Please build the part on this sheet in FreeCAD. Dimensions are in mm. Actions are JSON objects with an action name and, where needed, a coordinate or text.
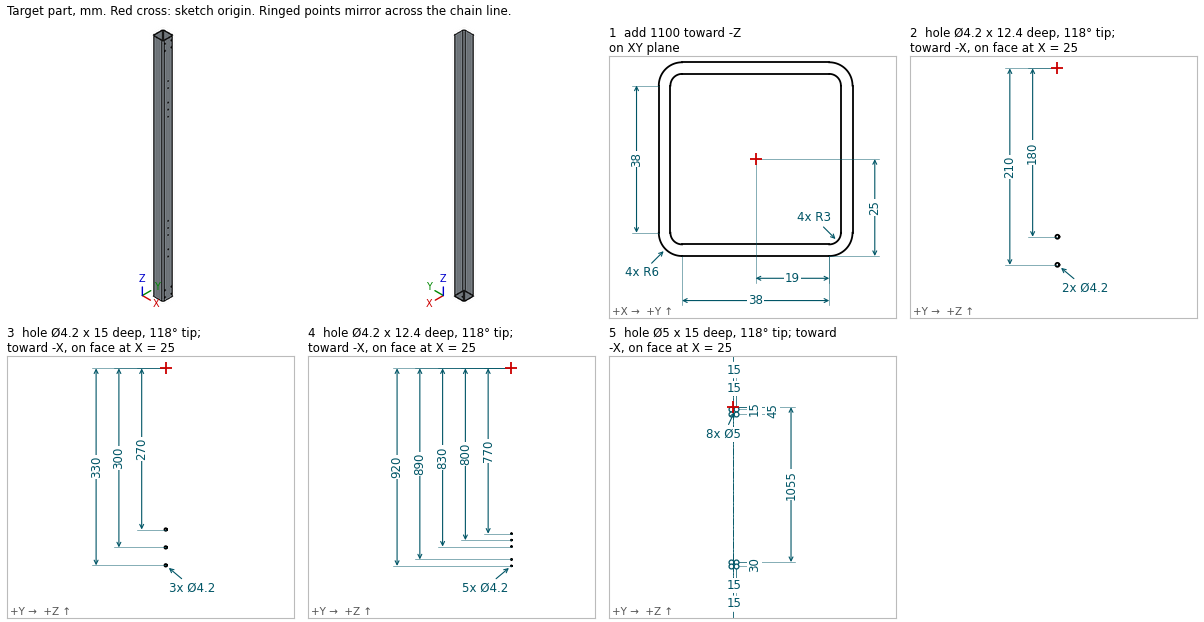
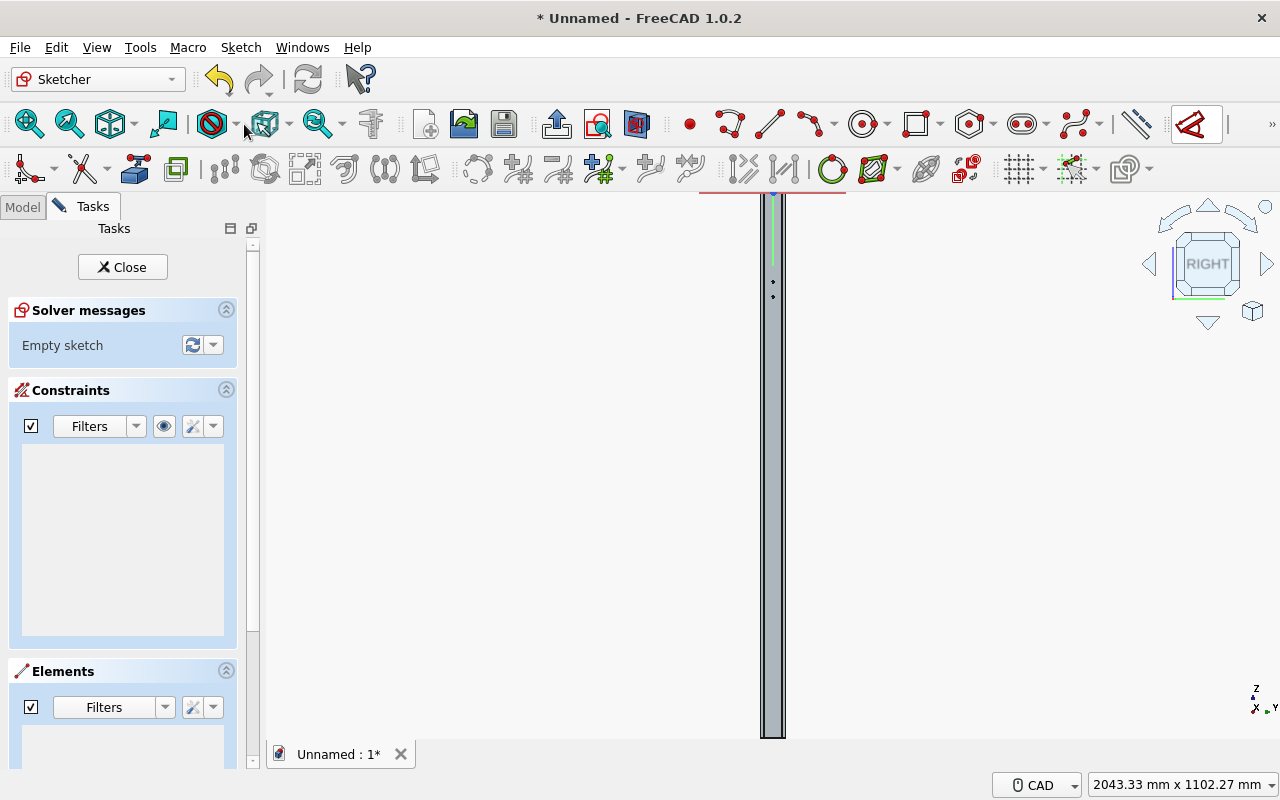
{"action": "scroll", "coordinate": [780, 329], "scroll_direction": "up", "scroll_amount": 12}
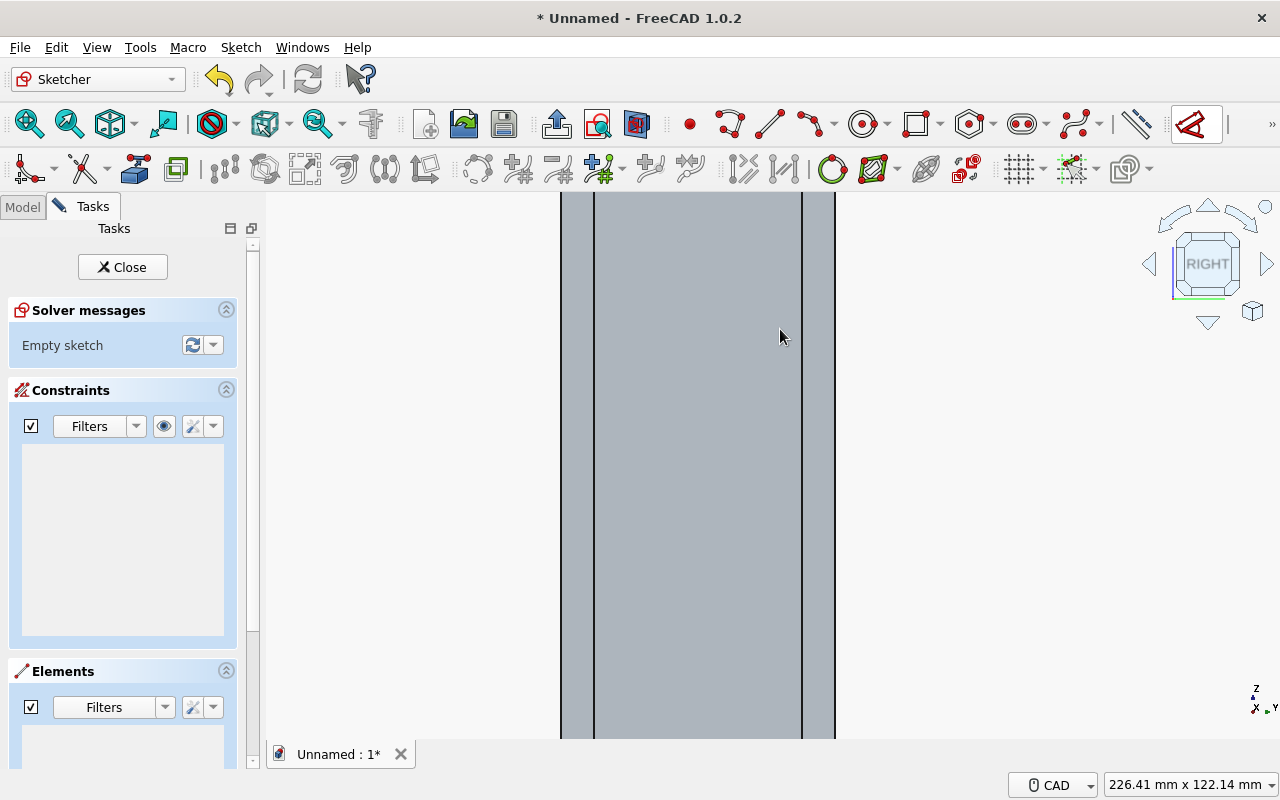
{"action": "left_click", "coordinate": [864, 124]}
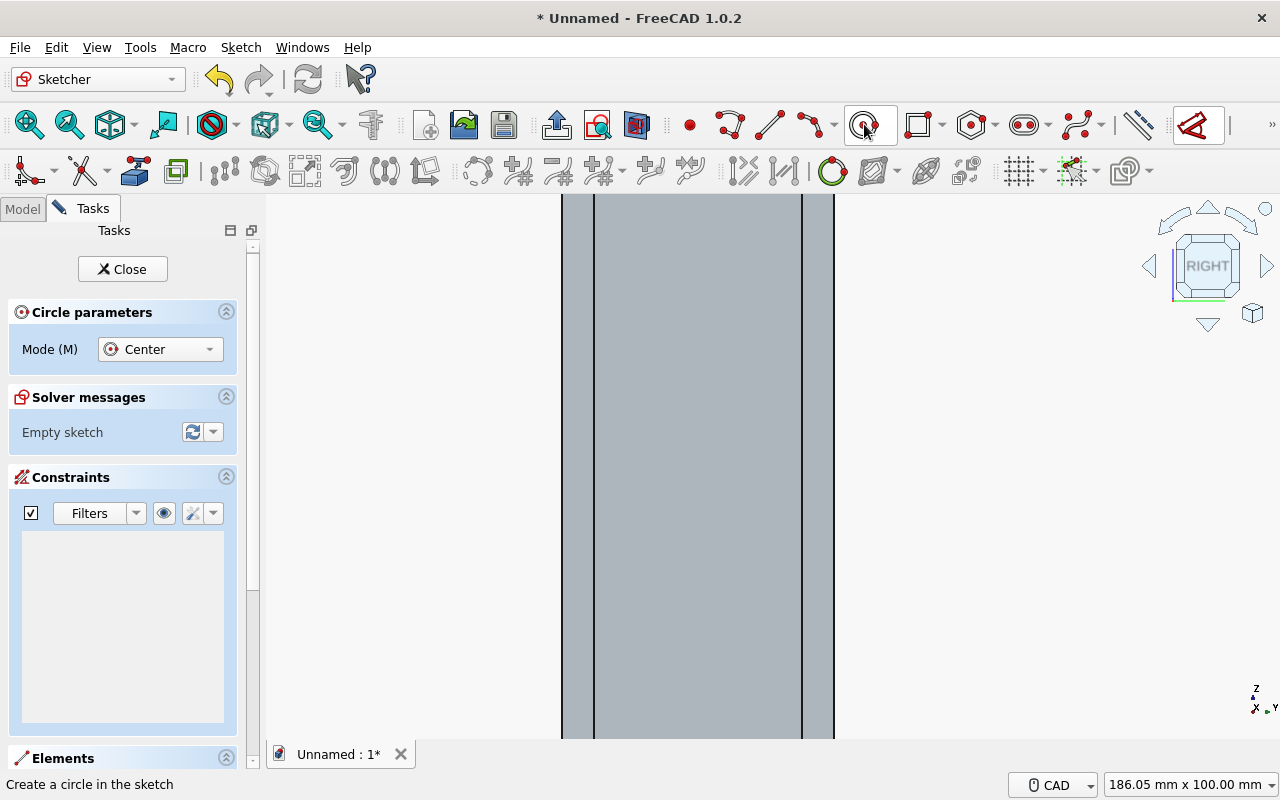
{"action": "scroll", "coordinate": [698, 301], "scroll_direction": "up", "scroll_amount": 4}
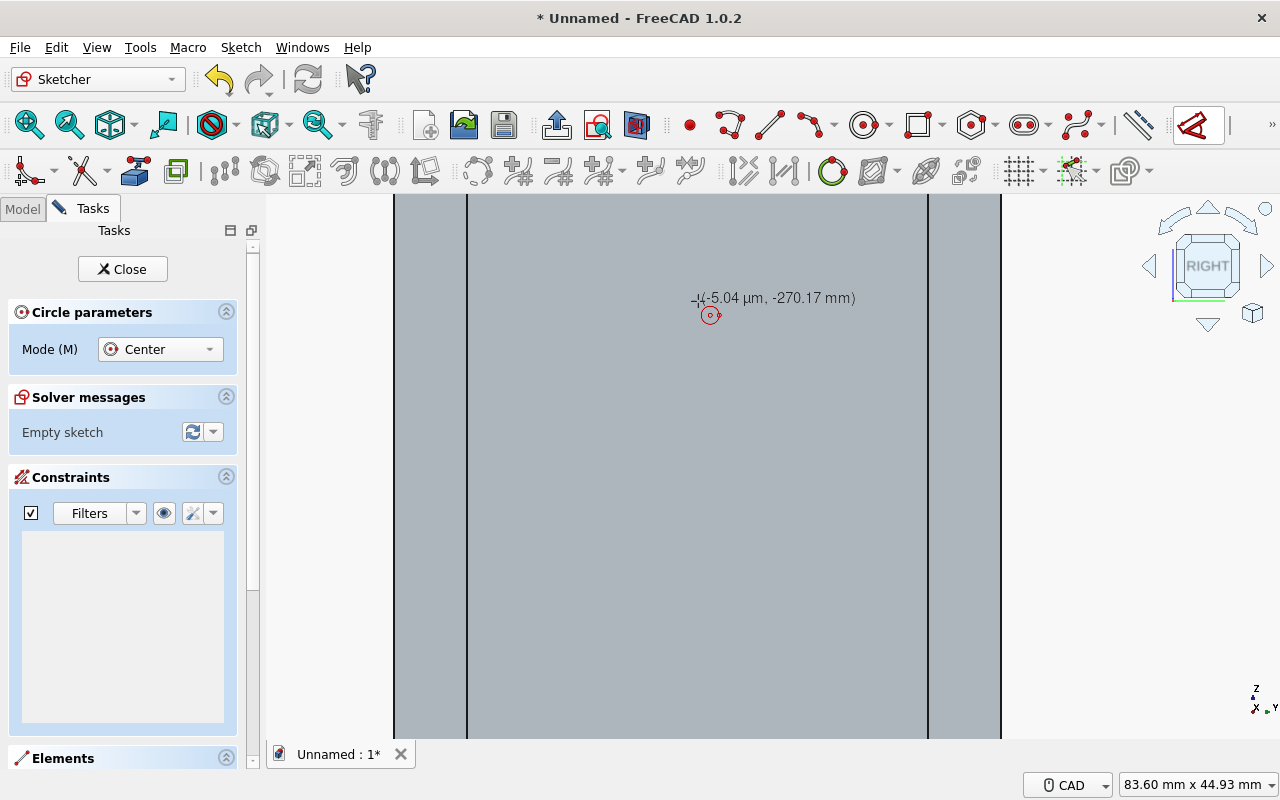
{"action": "left_click", "coordinate": [698, 301]}
{"action": "mouse_move", "coordinate": [716, 283]}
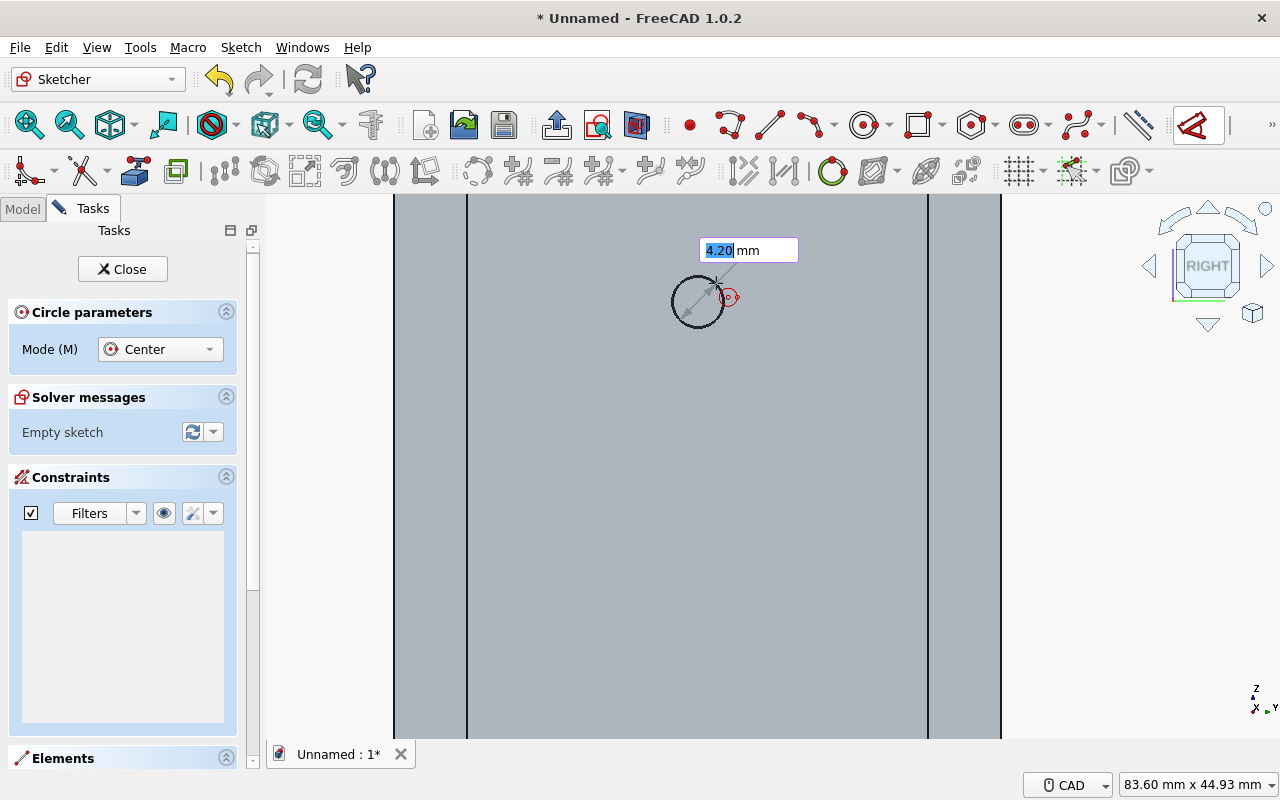
{"action": "type", "text": "4.2"}
{"action": "key", "text": "Return"}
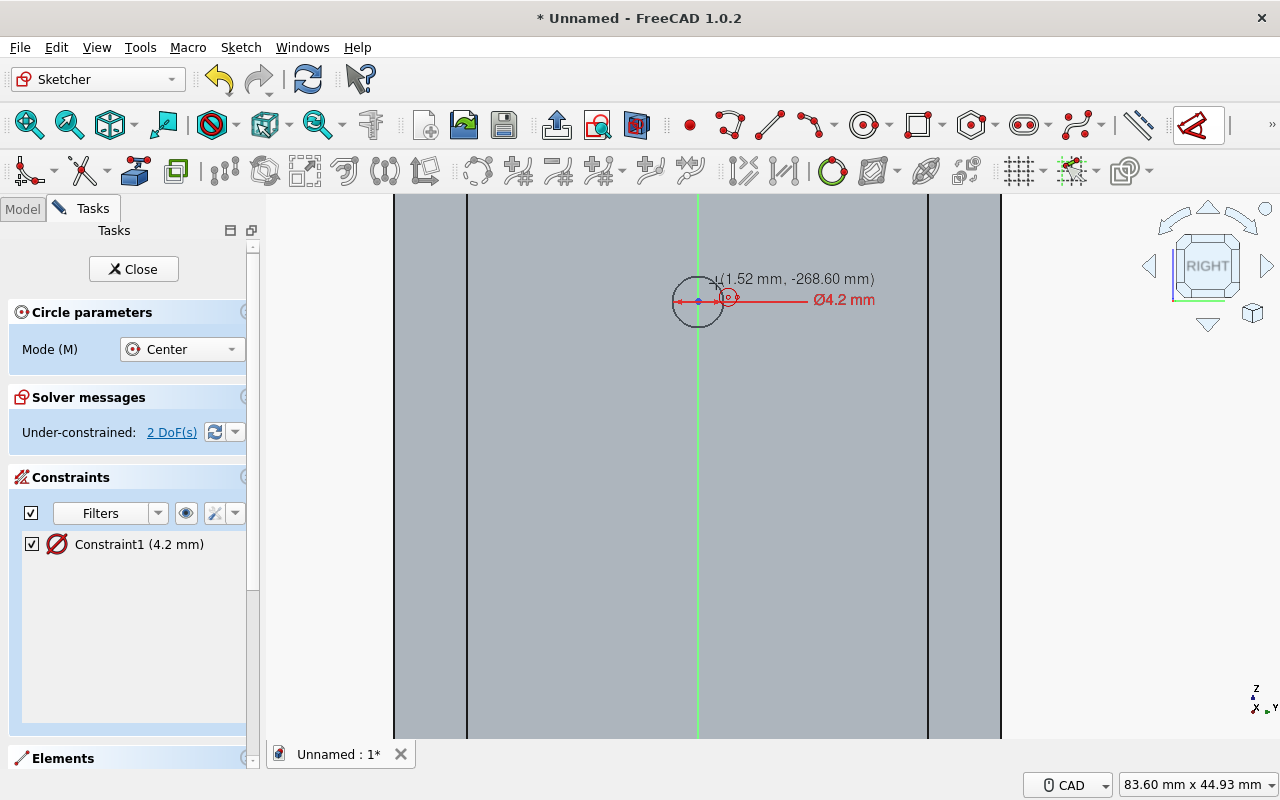
{"action": "left_click", "coordinate": [698, 665]}
{"action": "mouse_move", "coordinate": [716, 647]}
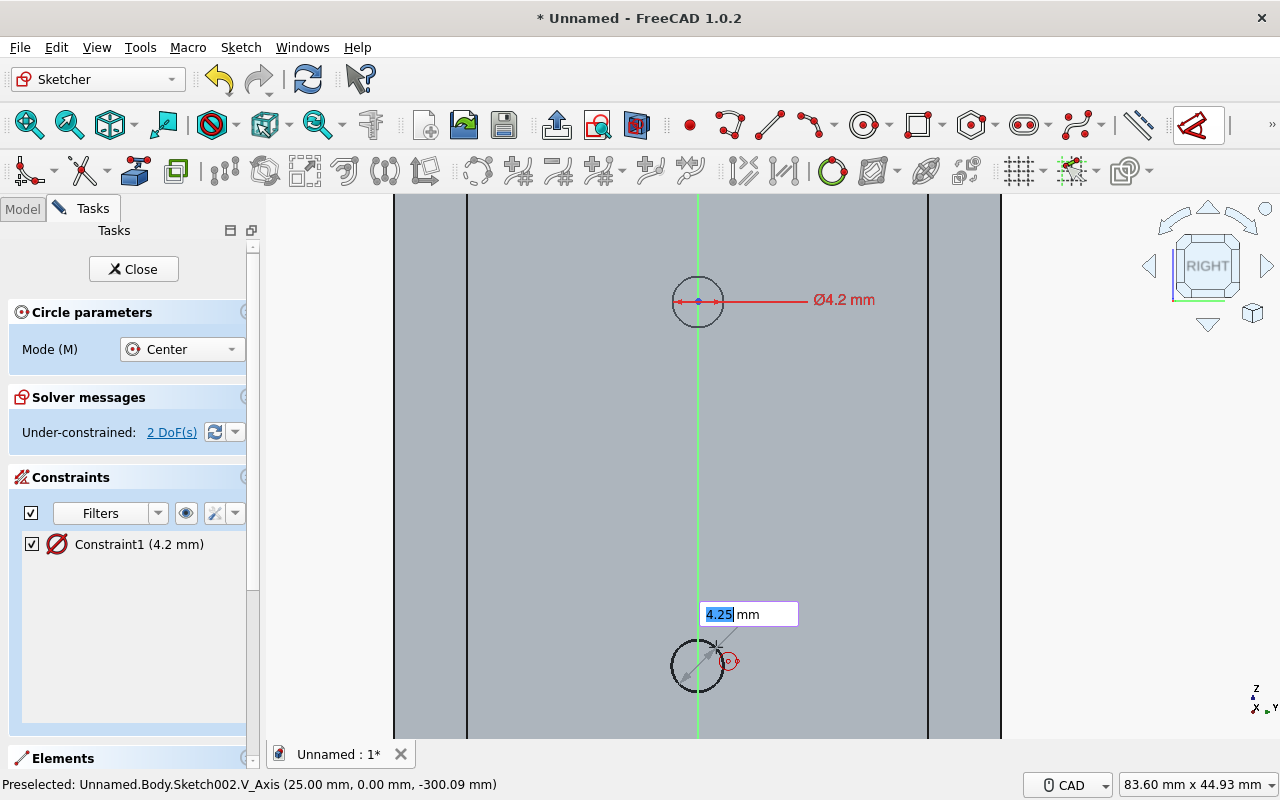
{"action": "type", "text": "4.2"}
{"action": "key", "text": "Return"}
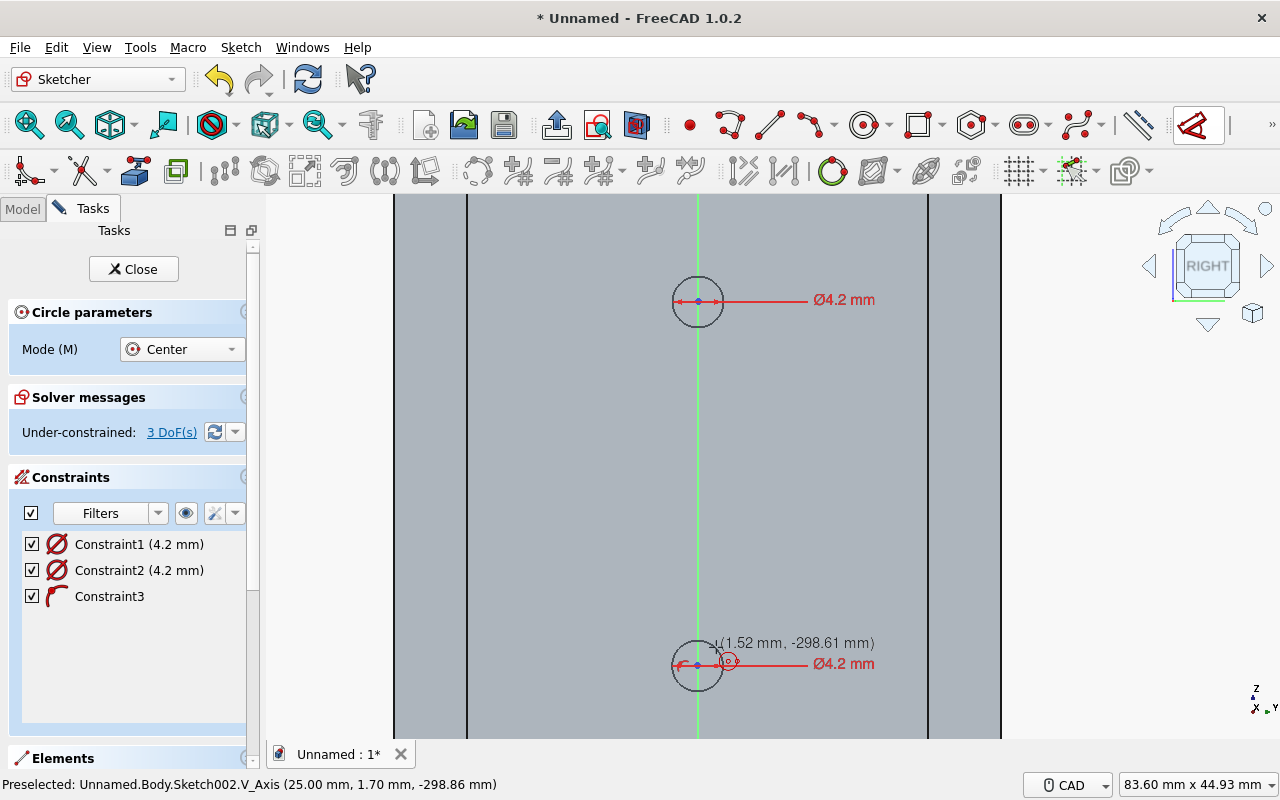
{"action": "scroll", "coordinate": [710, 305], "scroll_direction": "down", "scroll_amount": 4}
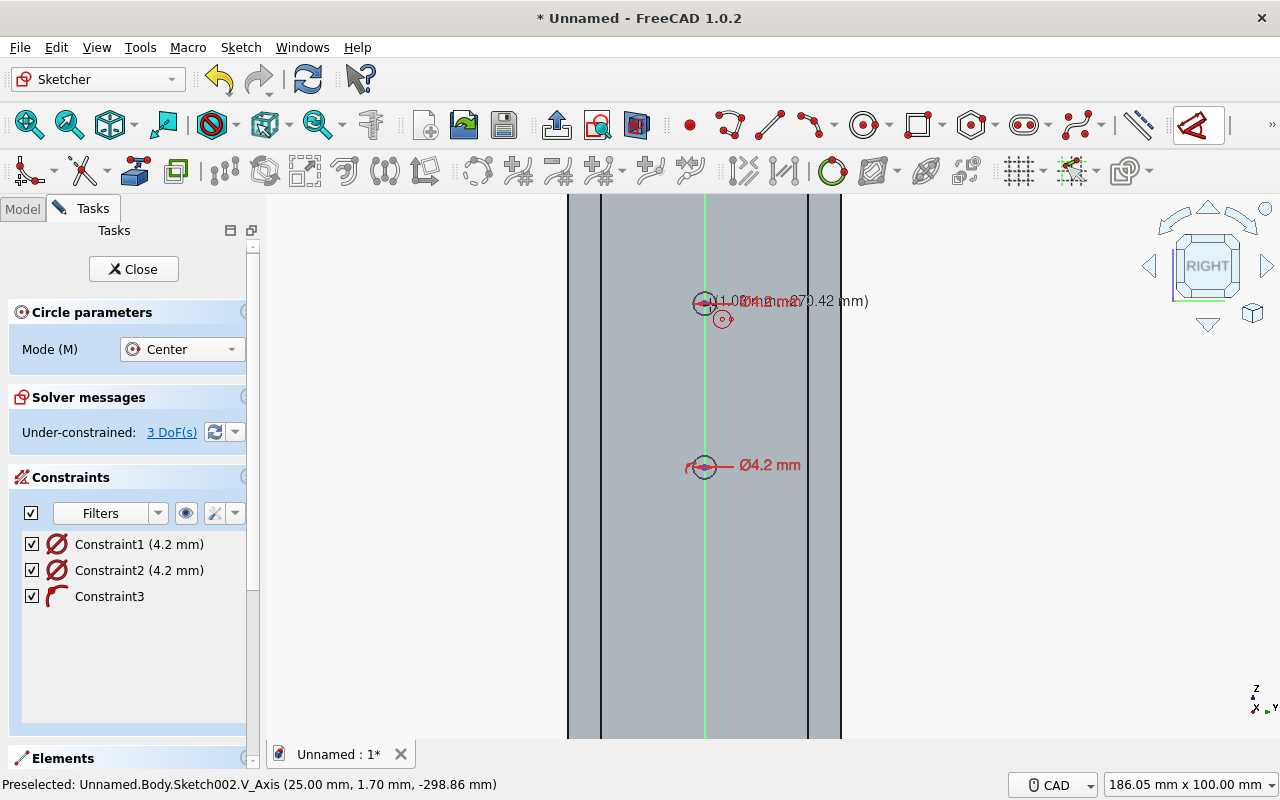
{"action": "scroll", "coordinate": [705, 630], "scroll_direction": "up", "scroll_amount": 4}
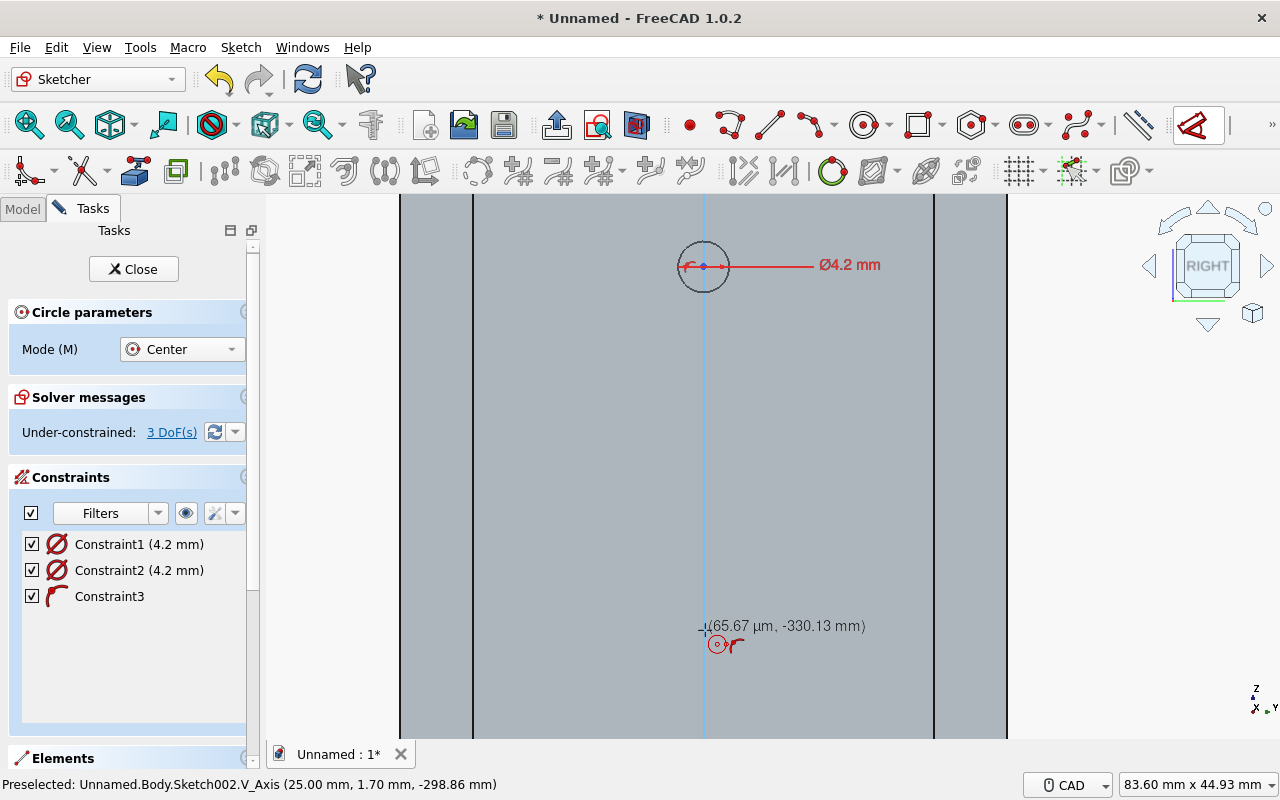
{"action": "left_click", "coordinate": [704, 630]}
{"action": "mouse_move", "coordinate": [722, 612]}